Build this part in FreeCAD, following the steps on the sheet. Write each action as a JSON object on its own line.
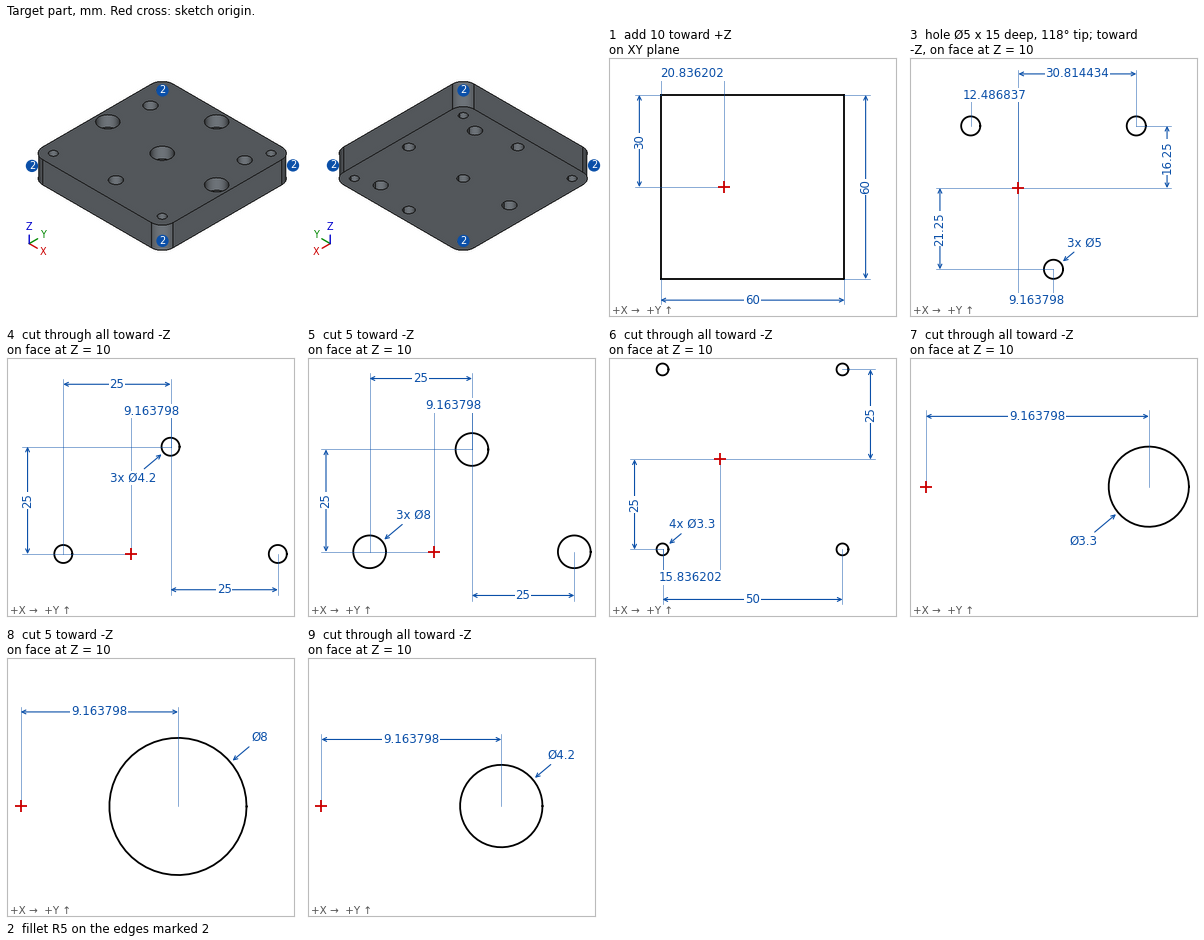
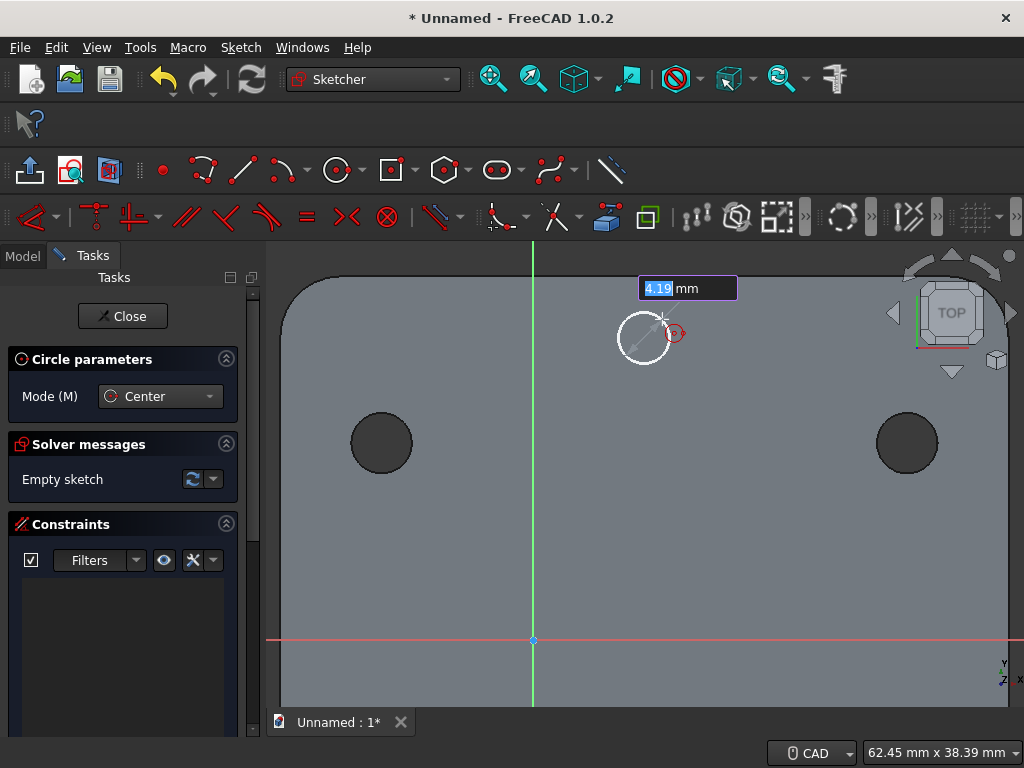
{"action": "type", "text": "4.2"}
{"action": "key", "text": "Return"}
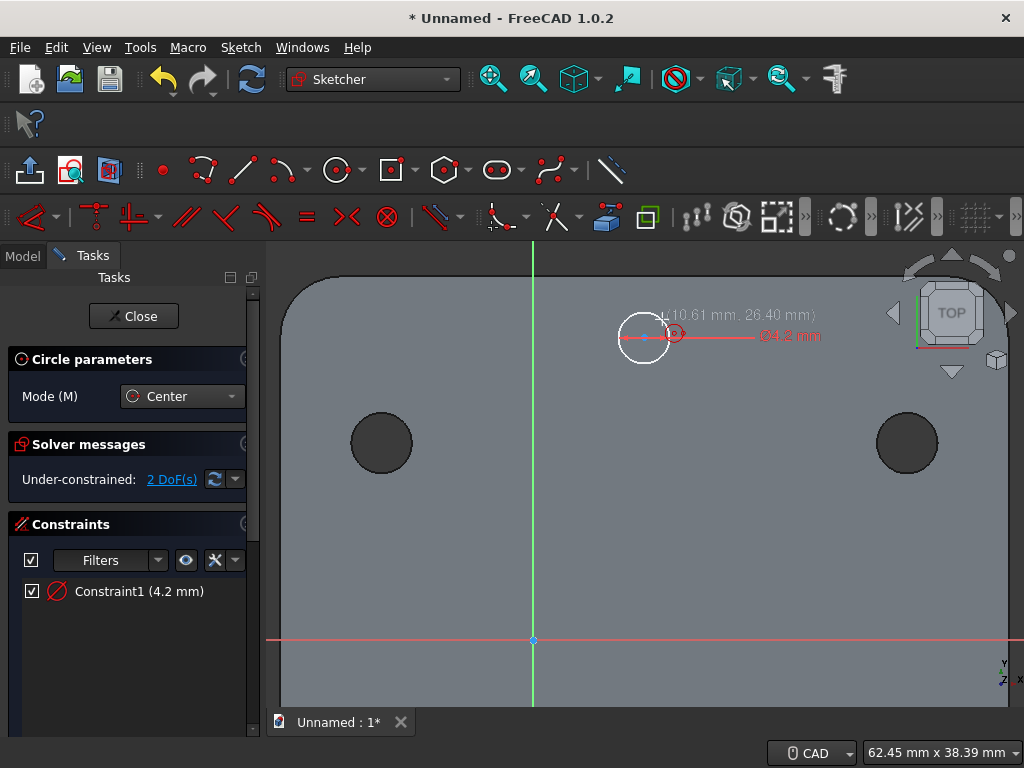
{"action": "scroll", "coordinate": [494, 456], "scroll_direction": "down", "scroll_amount": 3}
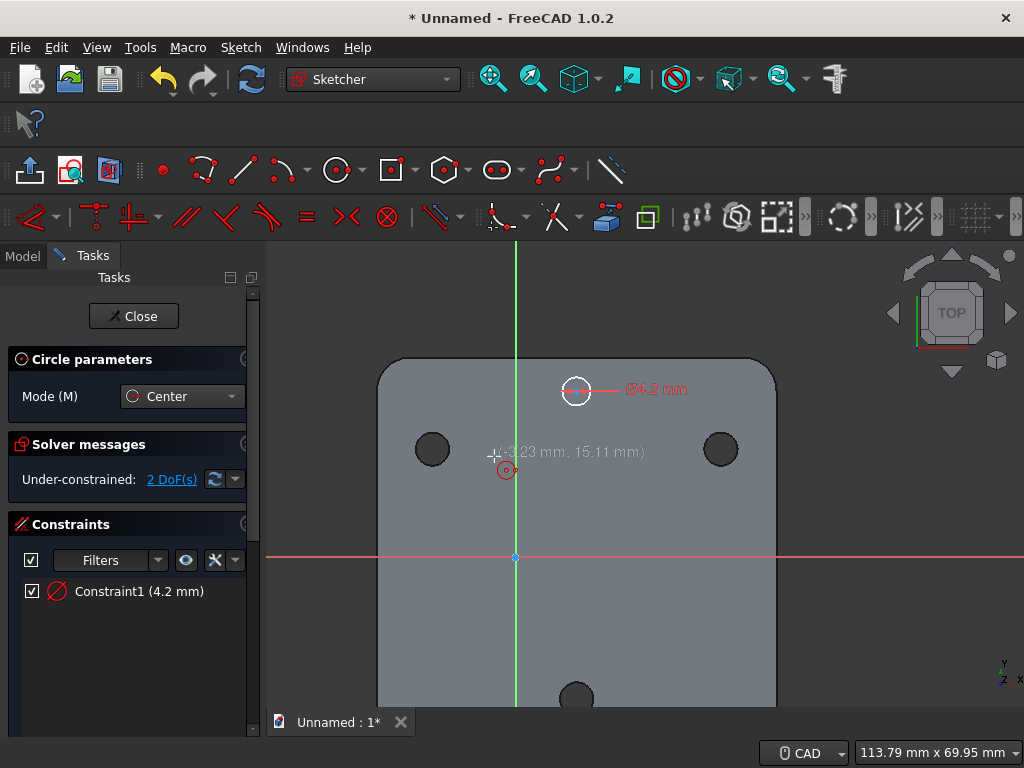
{"action": "scroll", "coordinate": [743, 557], "scroll_direction": "up", "scroll_amount": 3}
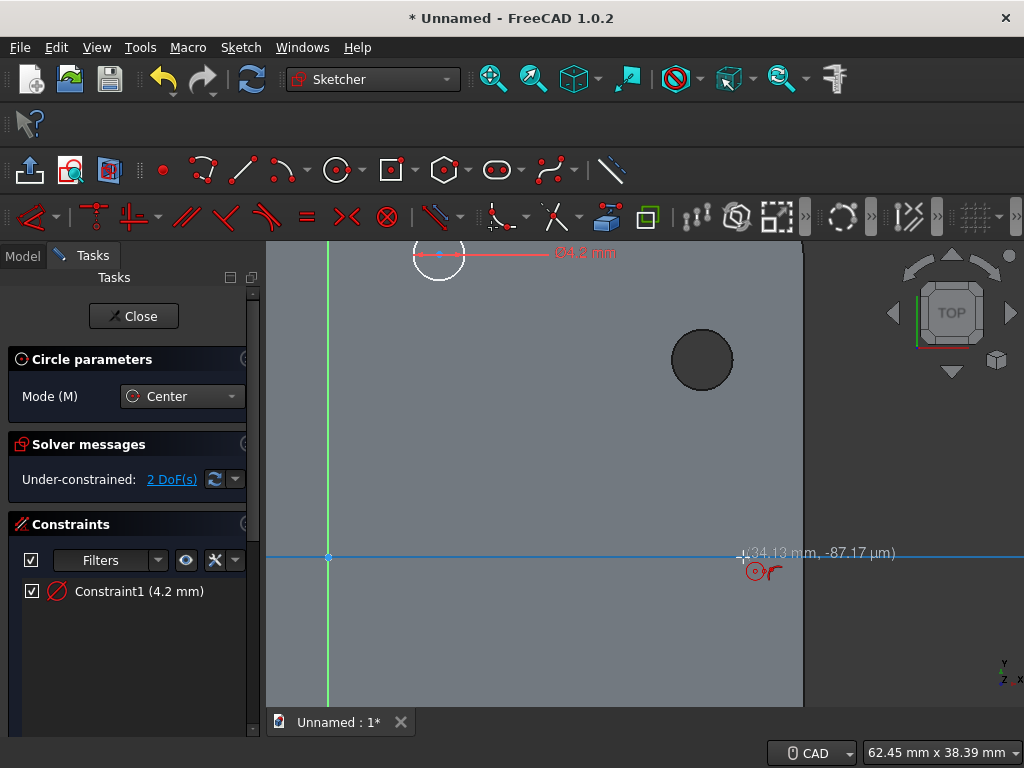
{"action": "left_click", "coordinate": [743, 557]}
{"action": "mouse_move", "coordinate": [761, 539]}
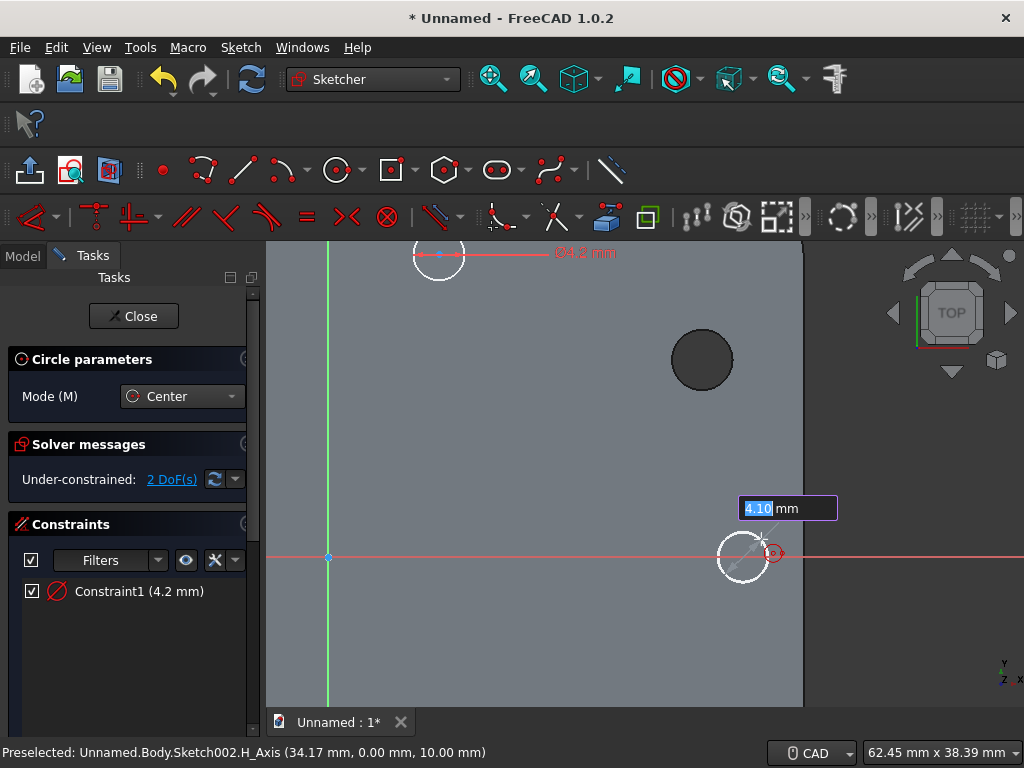
{"action": "type", "text": "4.2"}
{"action": "key", "text": "Return"}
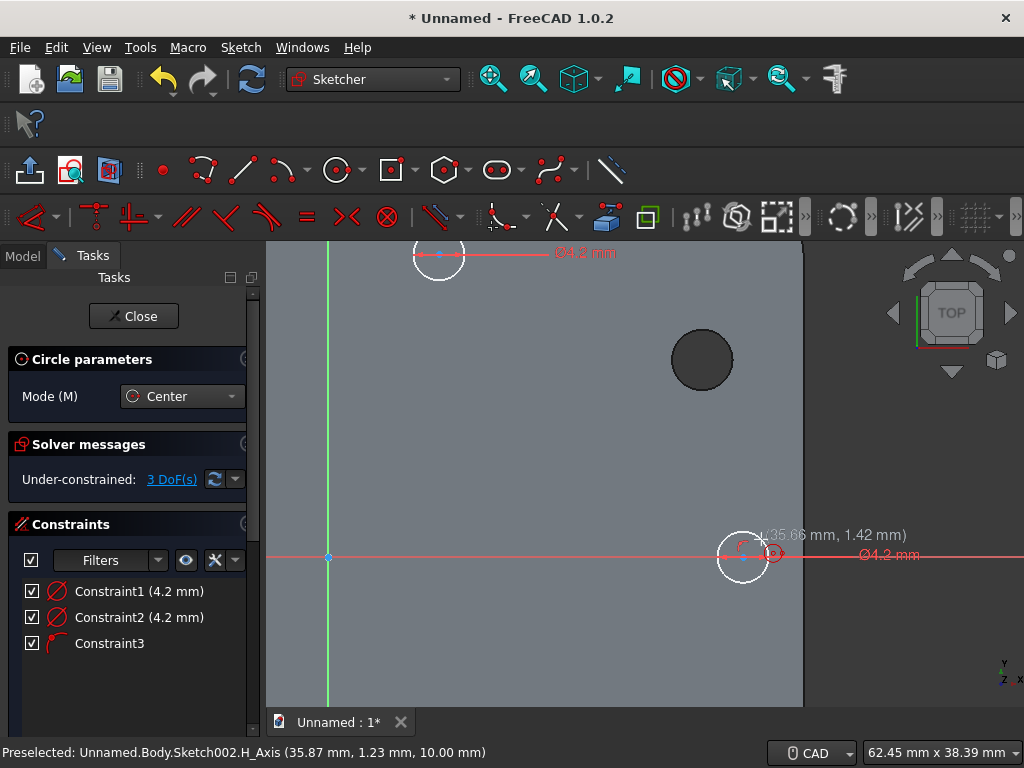
{"action": "scroll", "coordinate": [743, 557], "scroll_direction": "down", "scroll_amount": 3}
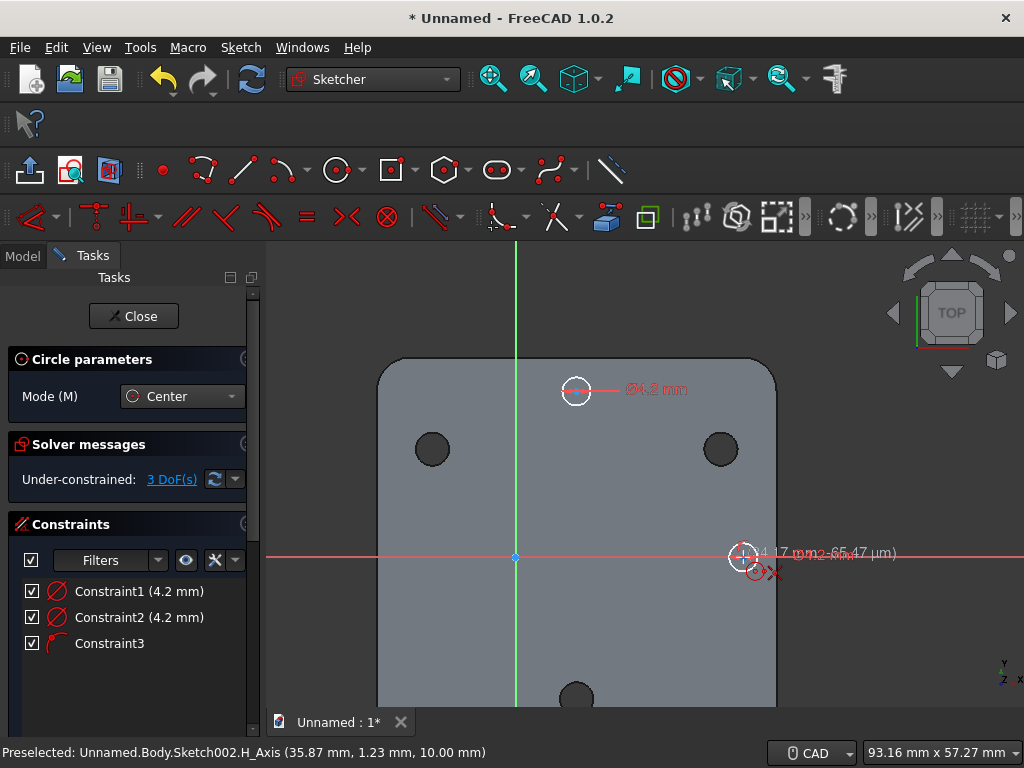
{"action": "scroll", "coordinate": [410, 557], "scroll_direction": "up", "scroll_amount": 3}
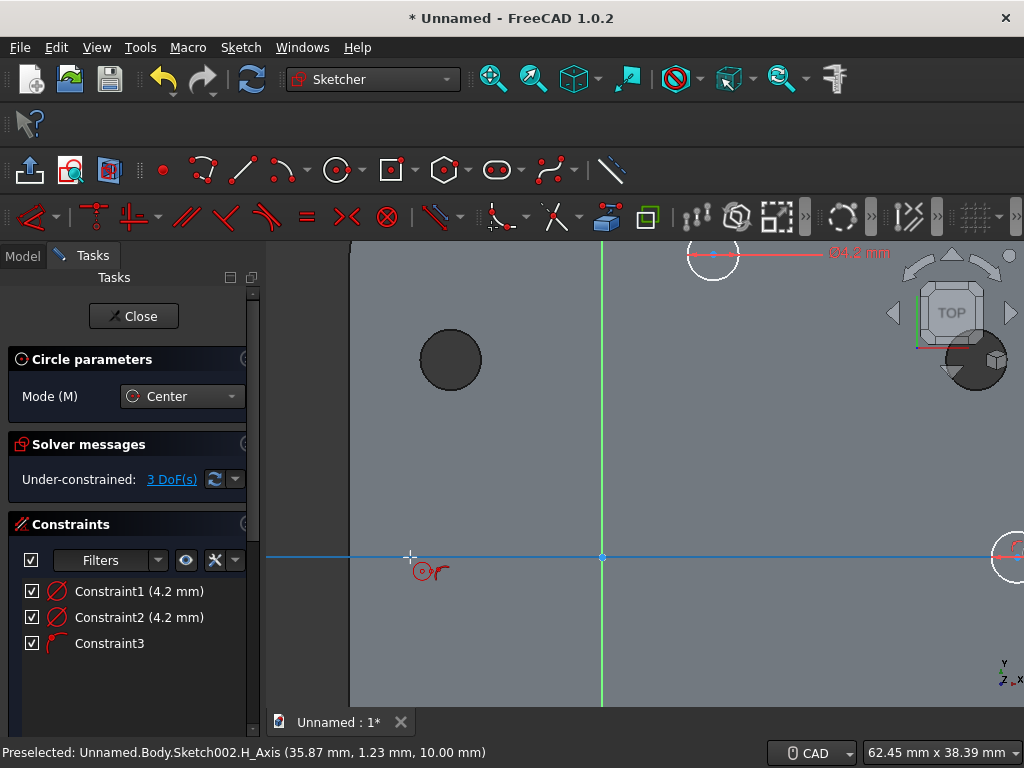
{"action": "left_click", "coordinate": [410, 557]}
{"action": "mouse_move", "coordinate": [428, 539]}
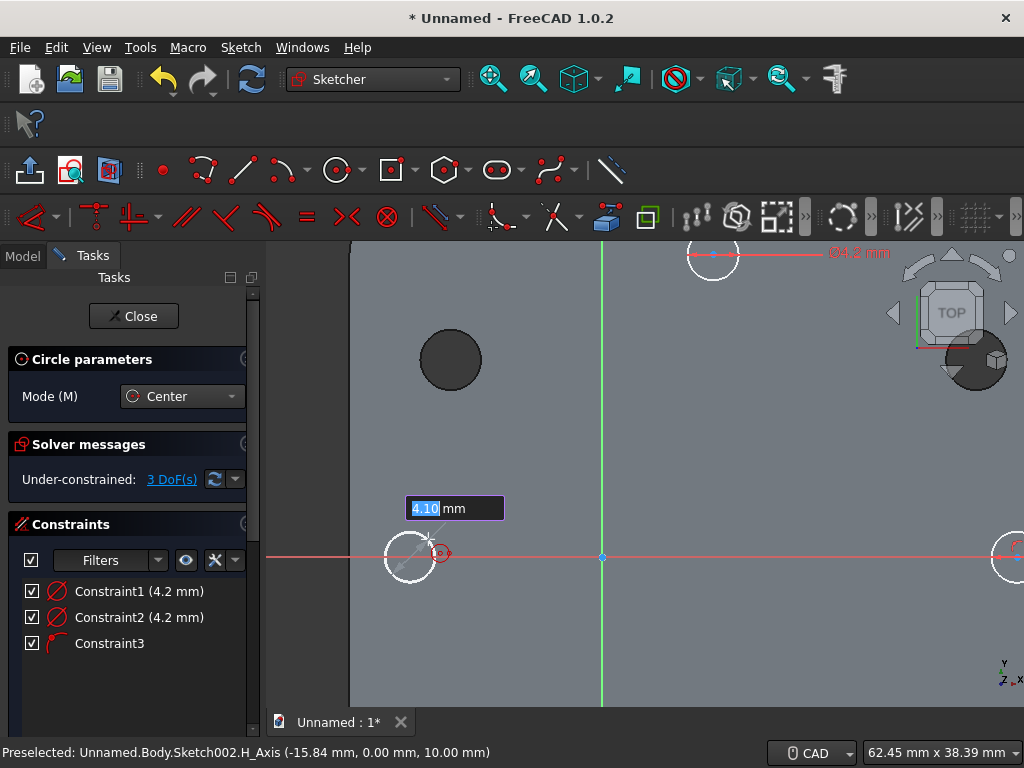
{"action": "type", "text": "4.2"}
{"action": "key", "text": "Return"}
{"action": "key", "text": "Escape"}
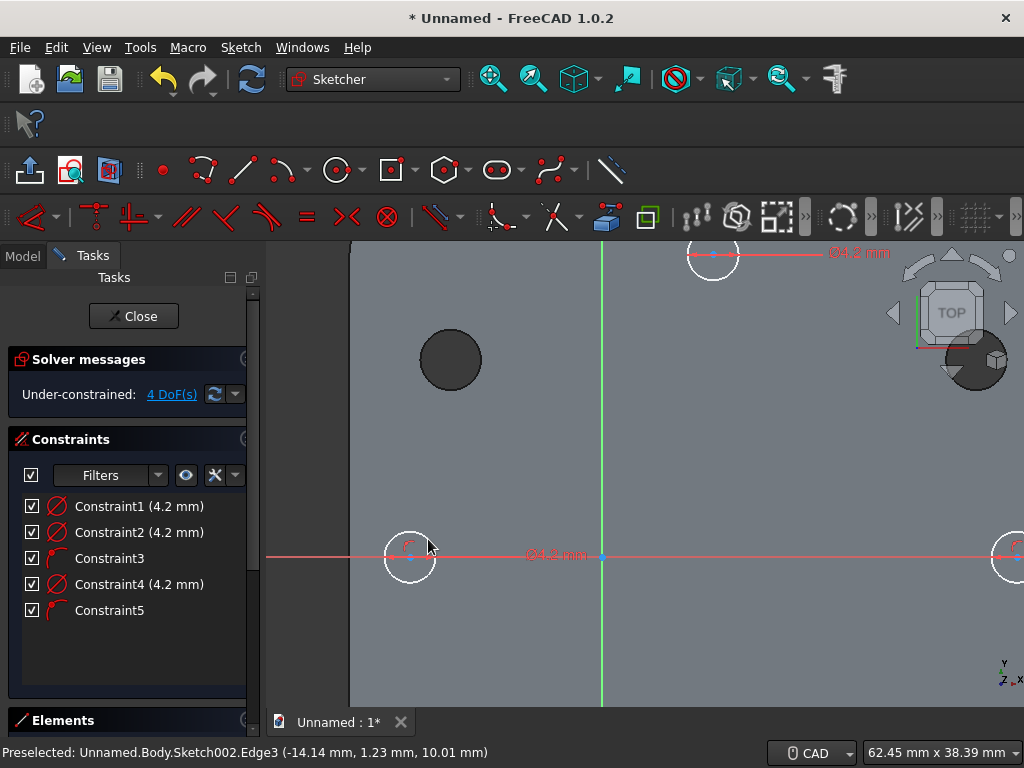
{"action": "left_click", "coordinate": [32, 218]}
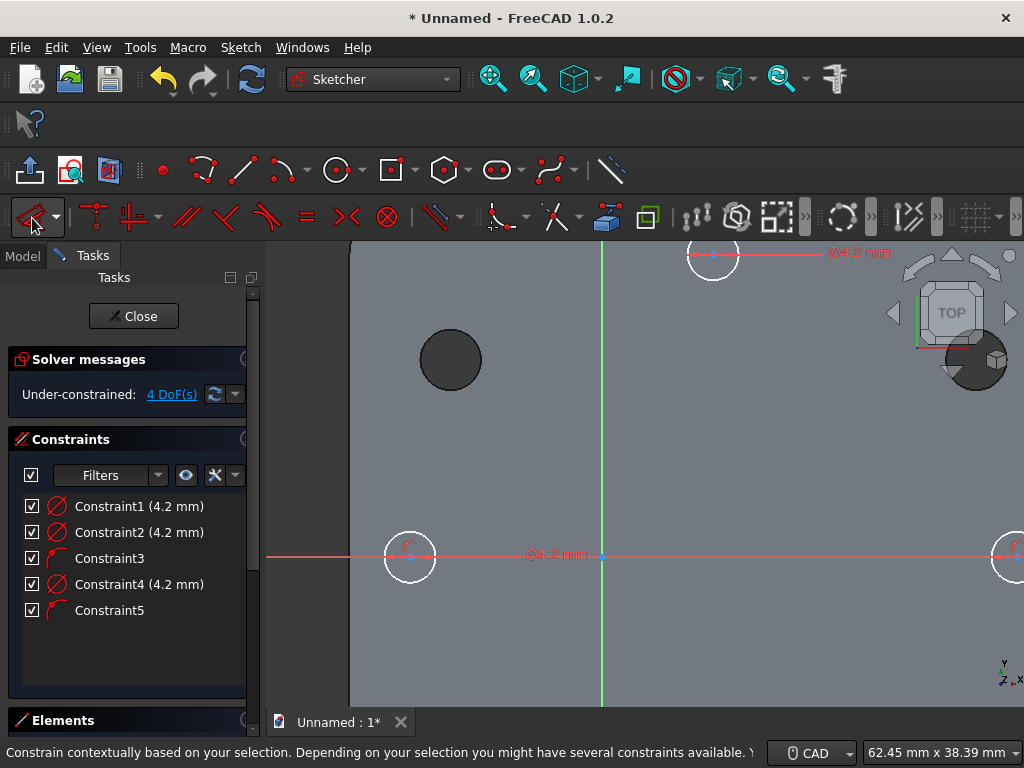
{"action": "scroll", "coordinate": [410, 557], "scroll_direction": "down", "scroll_amount": 3}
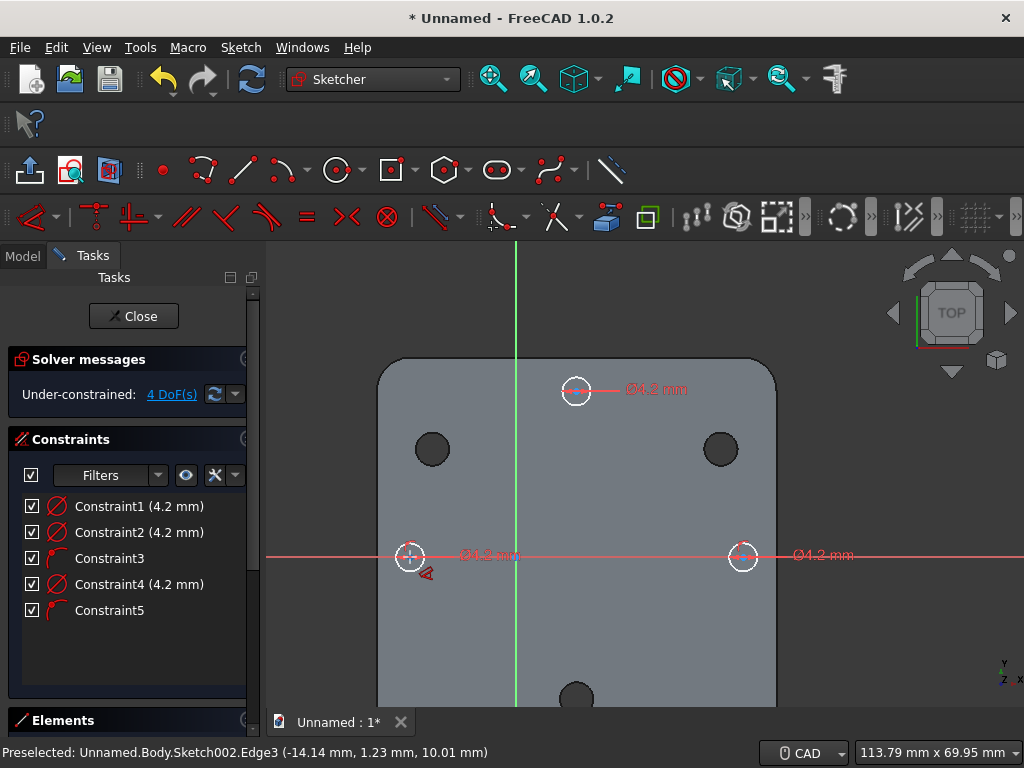
{"action": "left_click", "coordinate": [576, 391]}
{"action": "left_click", "coordinate": [482, 474]}